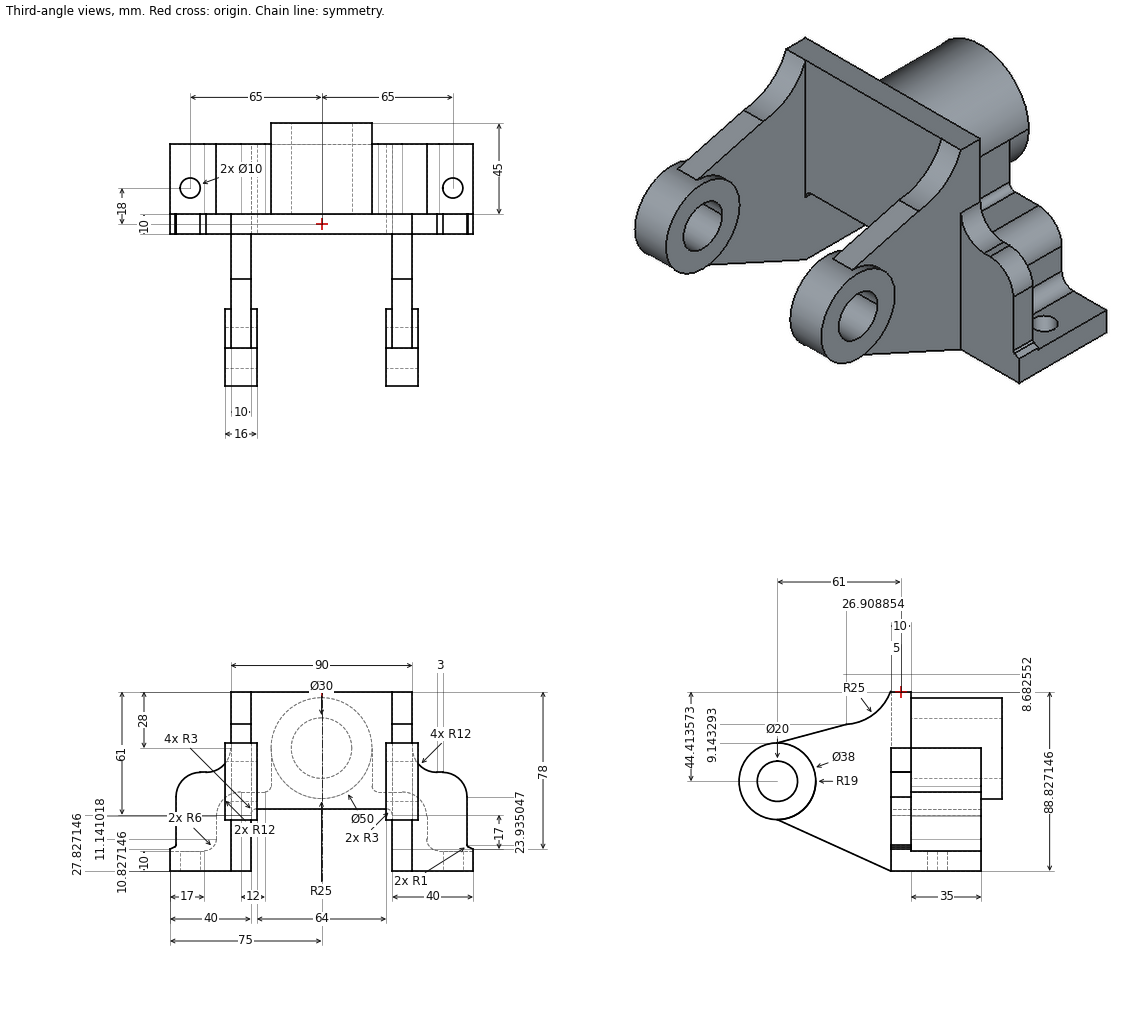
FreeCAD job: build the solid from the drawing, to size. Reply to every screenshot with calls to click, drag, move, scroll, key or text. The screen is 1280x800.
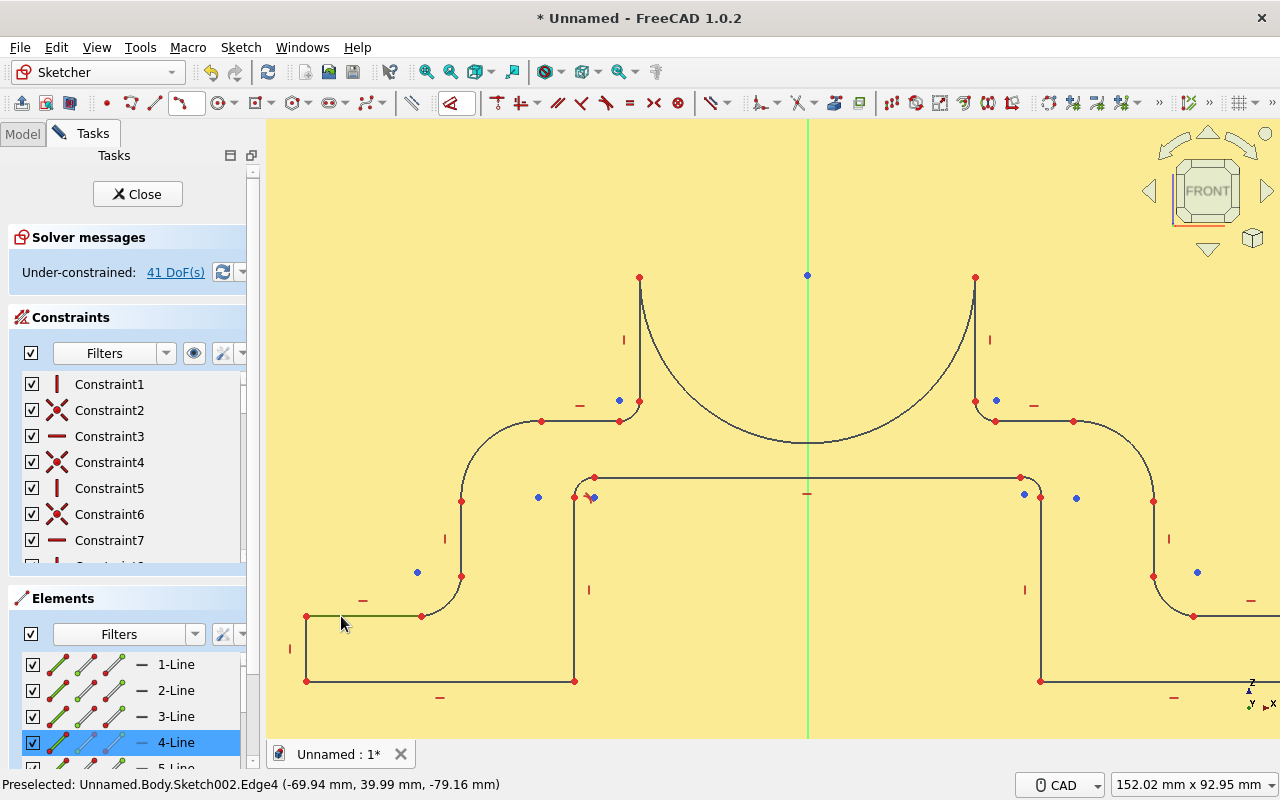
click(439, 611)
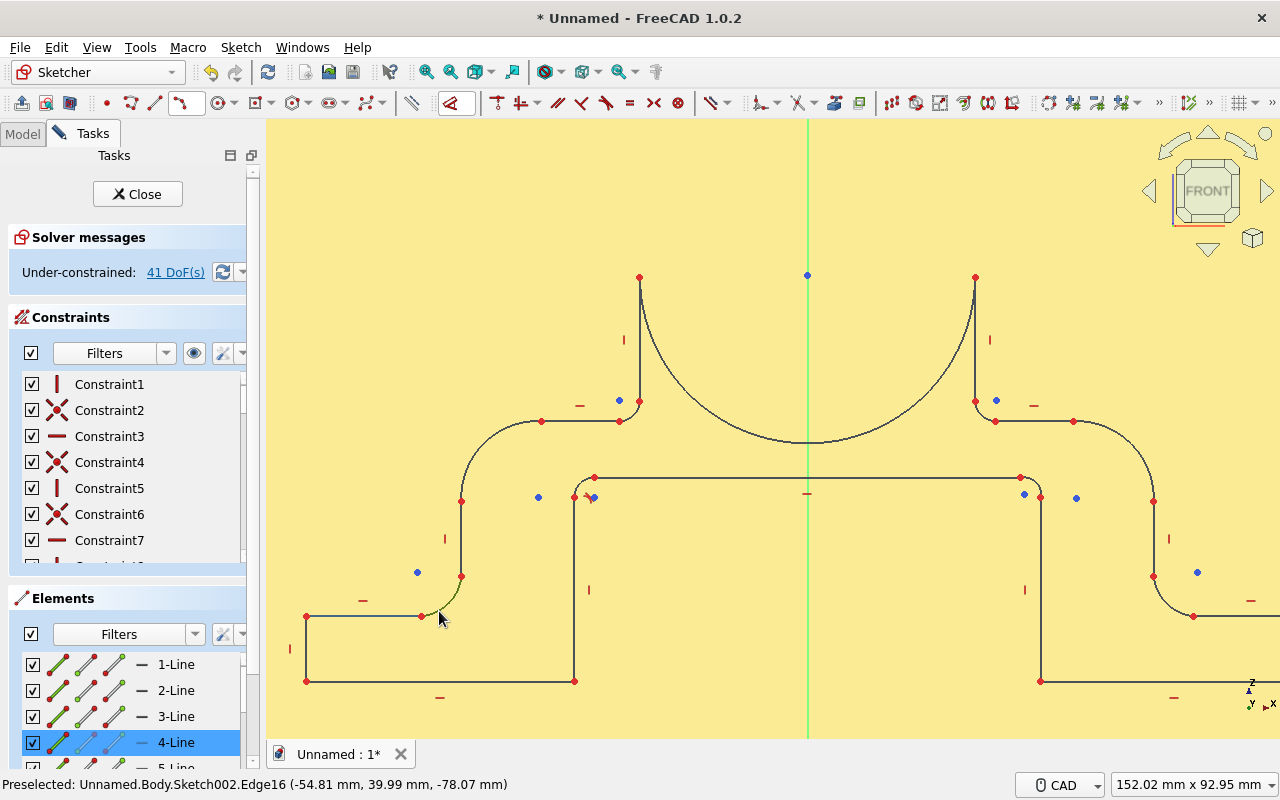
key(t)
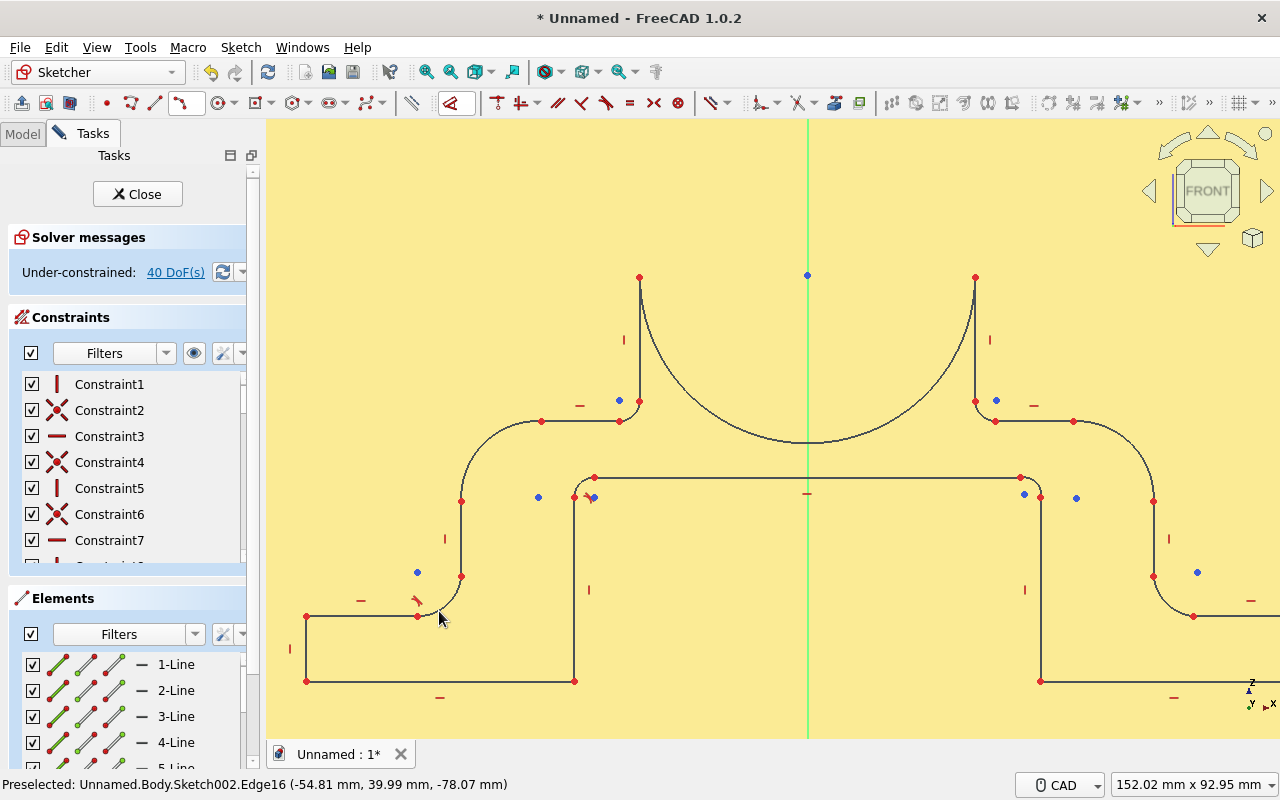
click(461, 554)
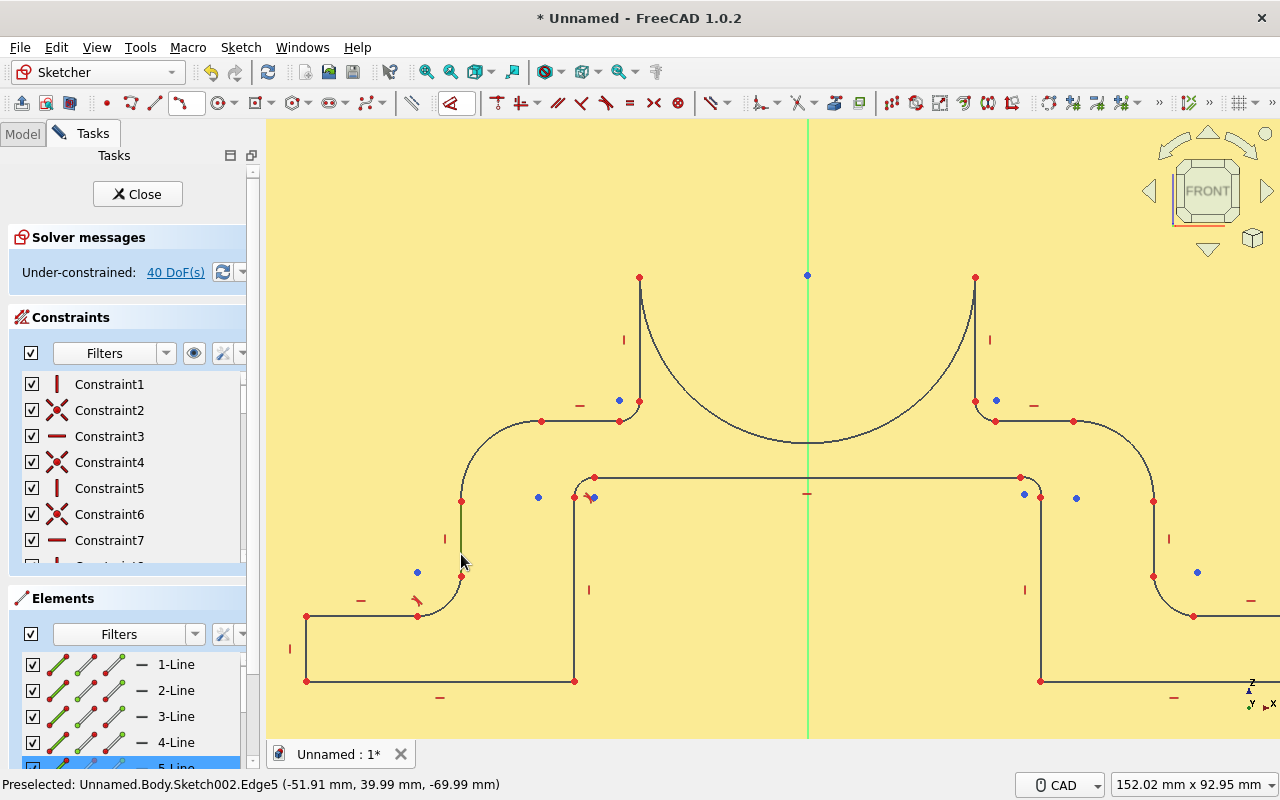
click(436, 612)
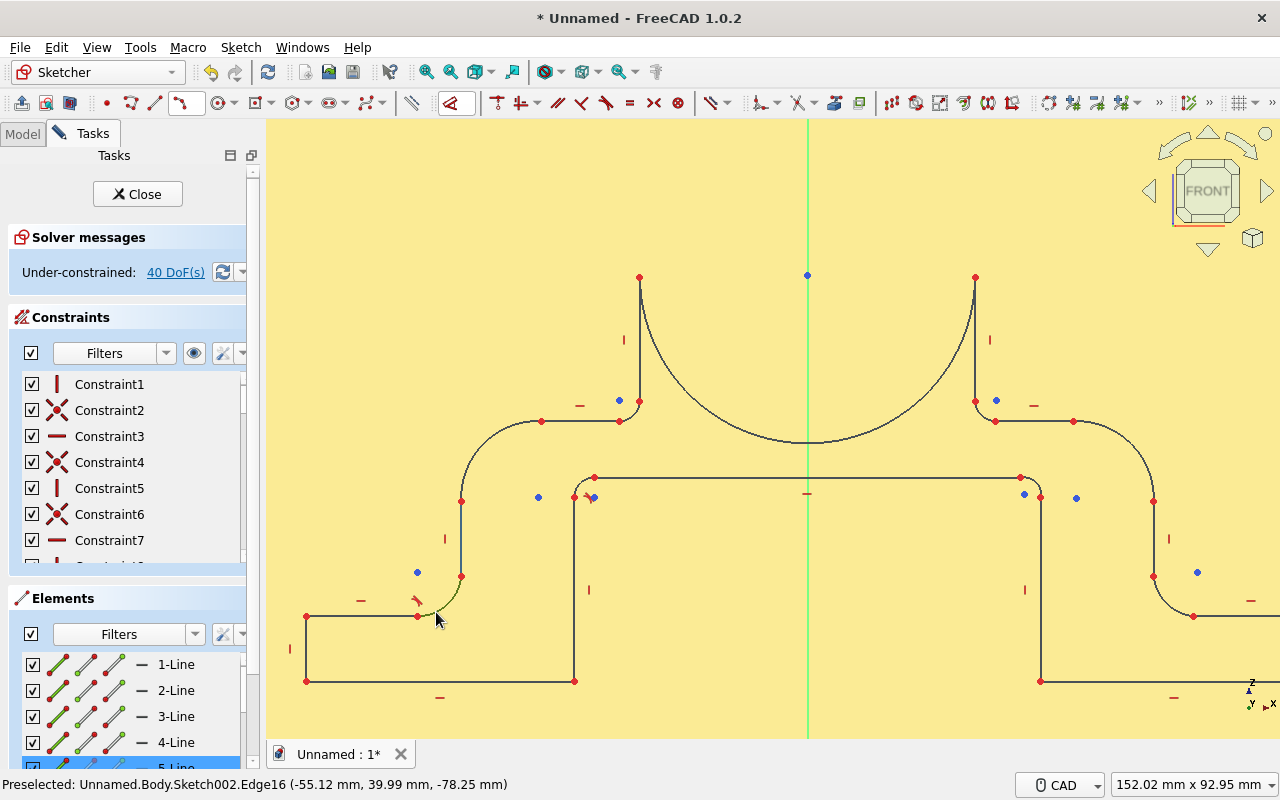
key(t)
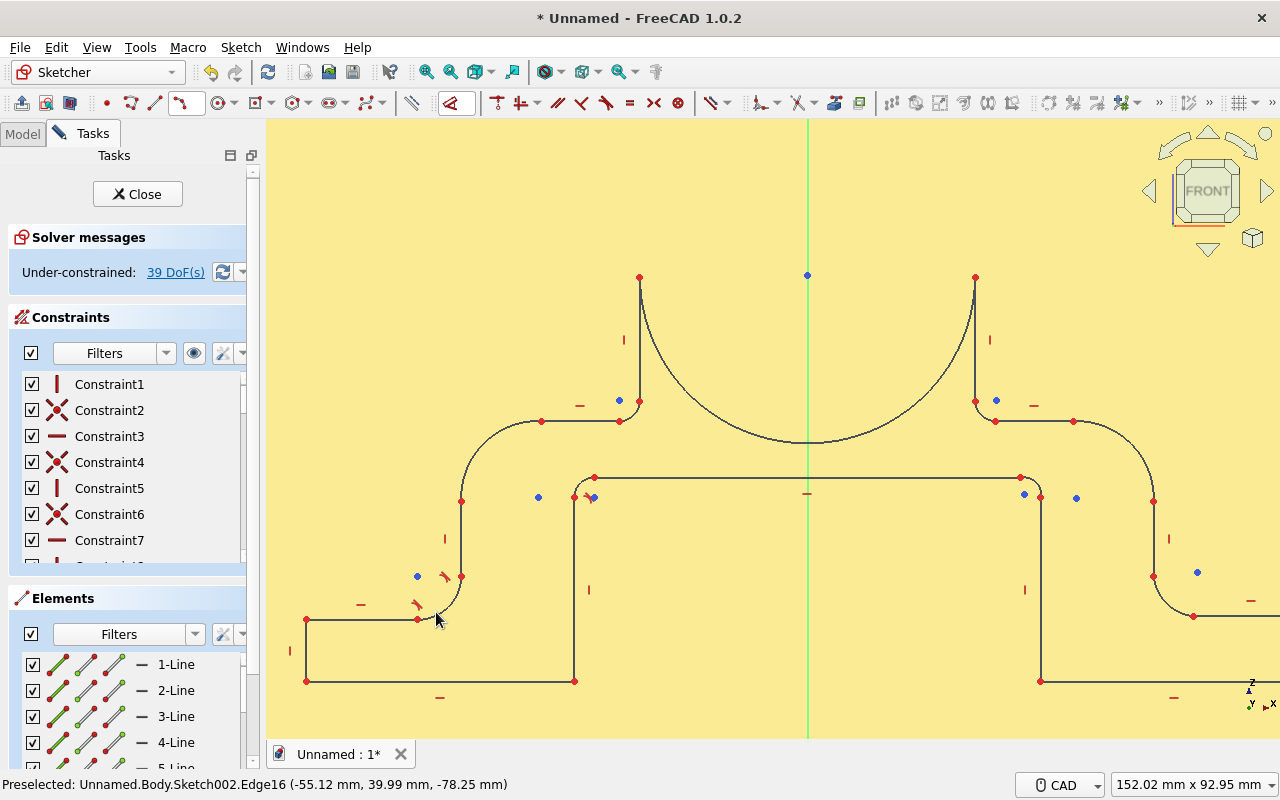
click(461, 554)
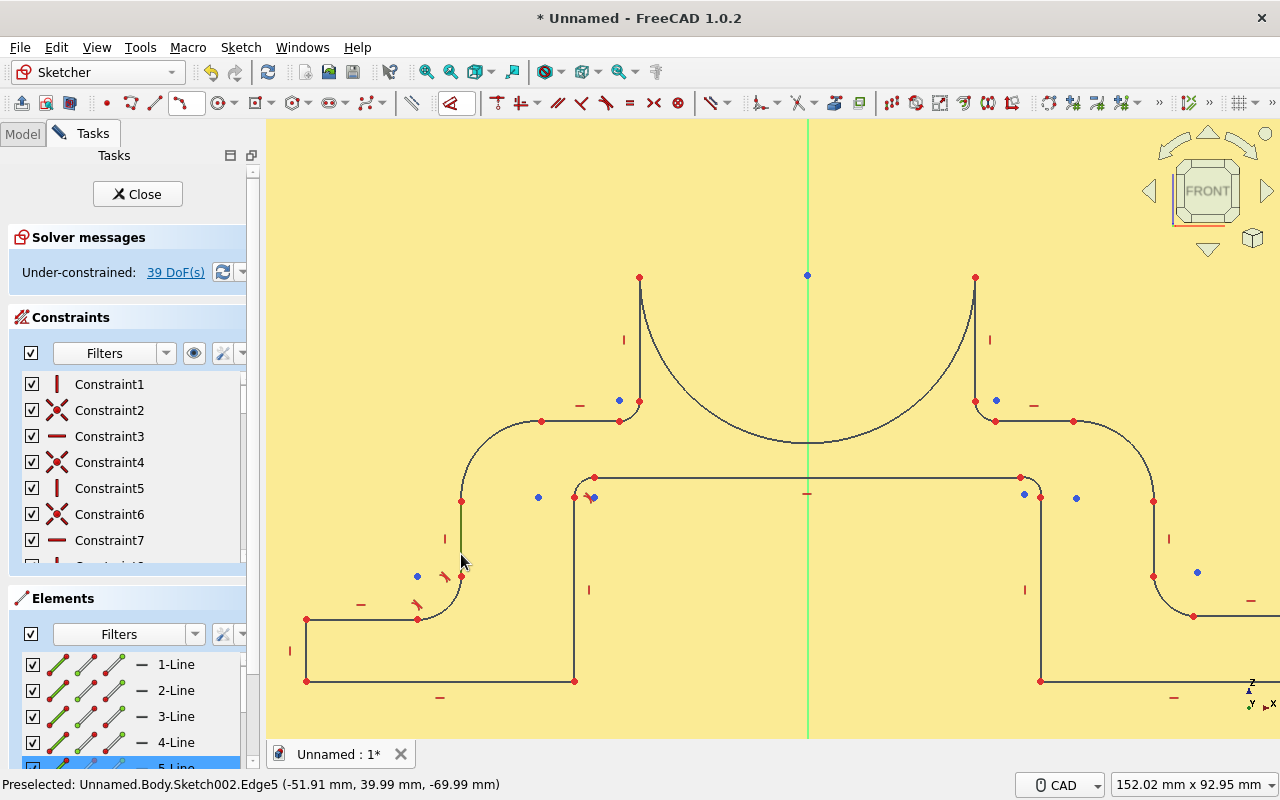
click(504, 429)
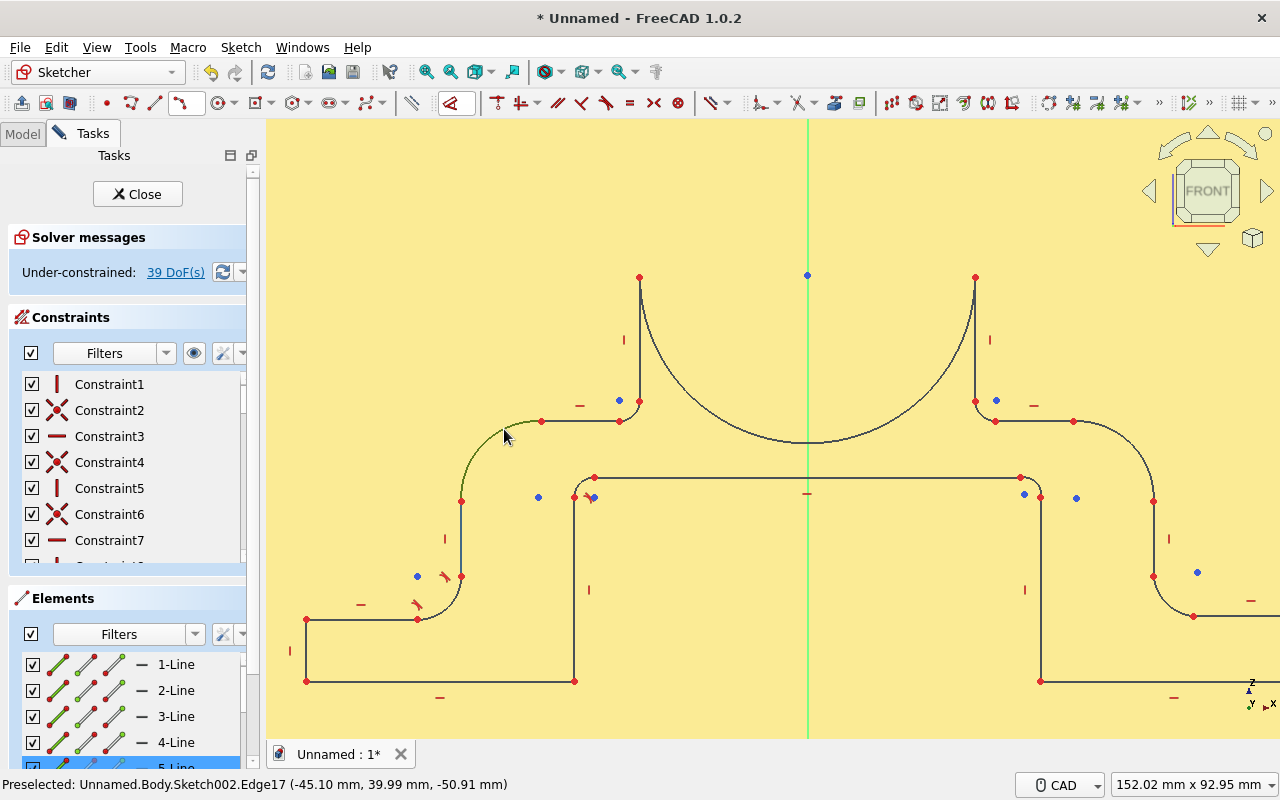
key(t)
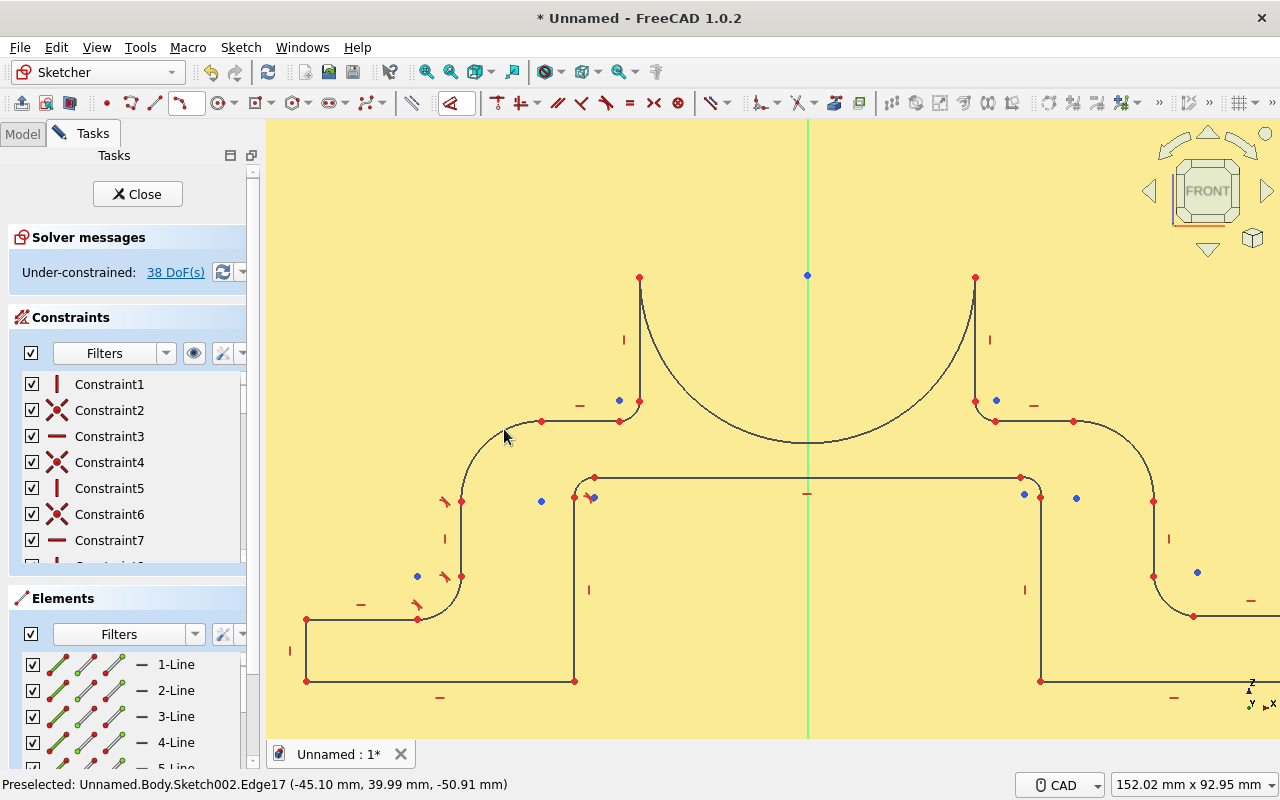
click(565, 421)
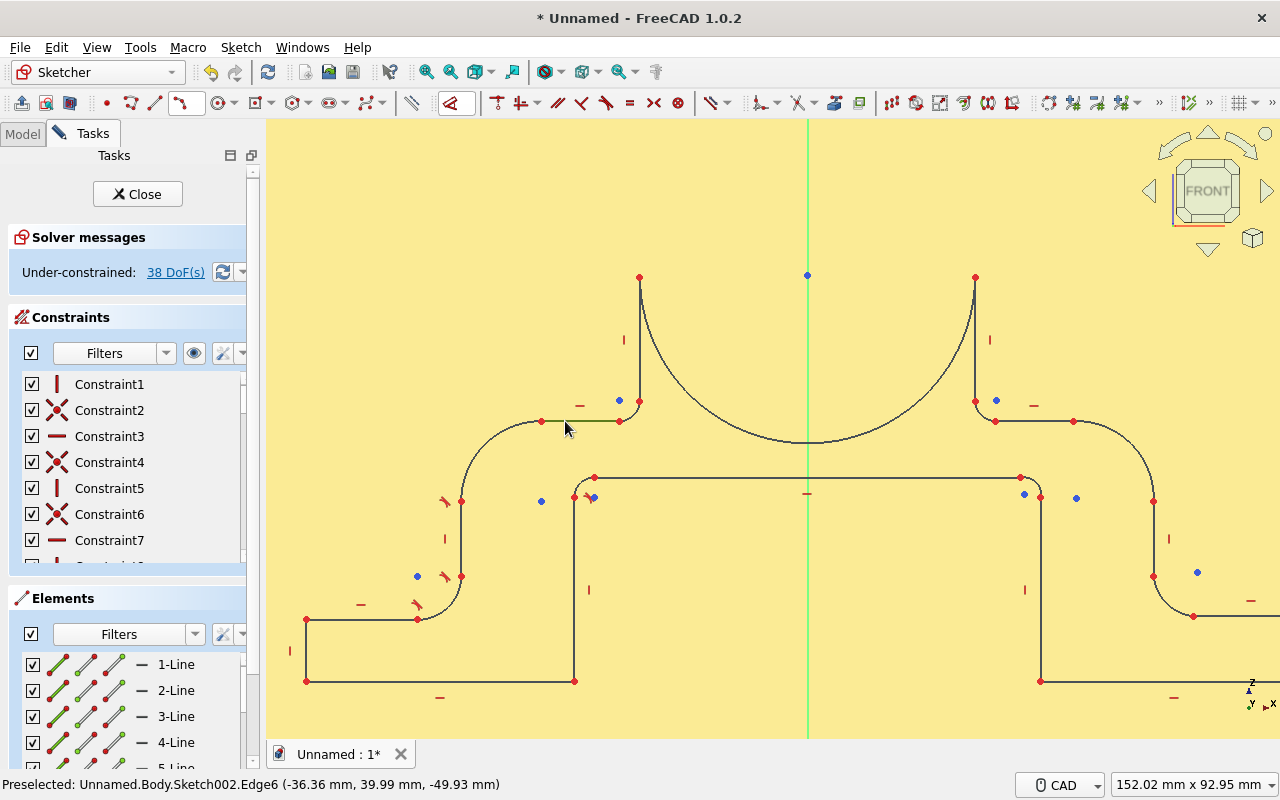
click(505, 430)